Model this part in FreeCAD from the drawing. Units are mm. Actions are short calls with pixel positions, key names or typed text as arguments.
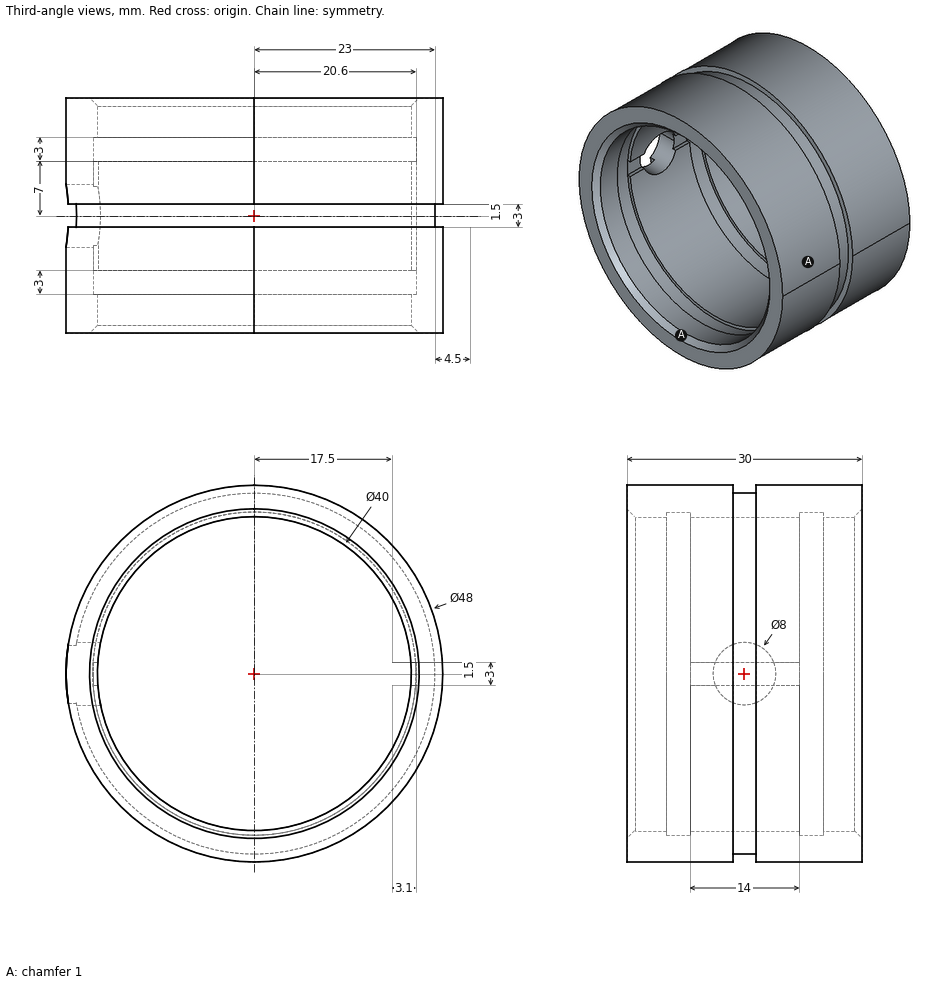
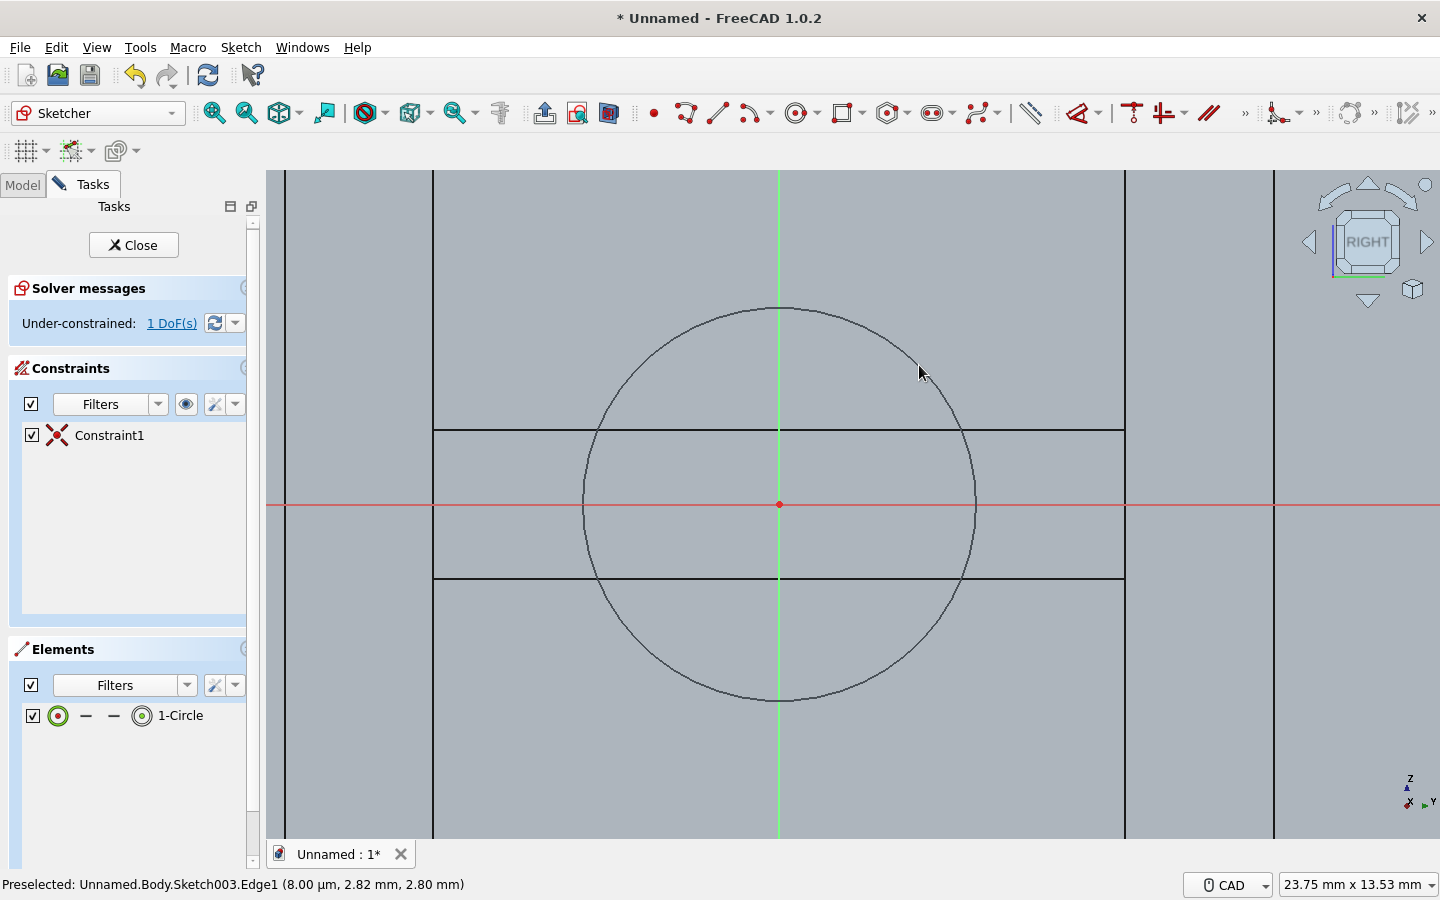
click(1078, 114)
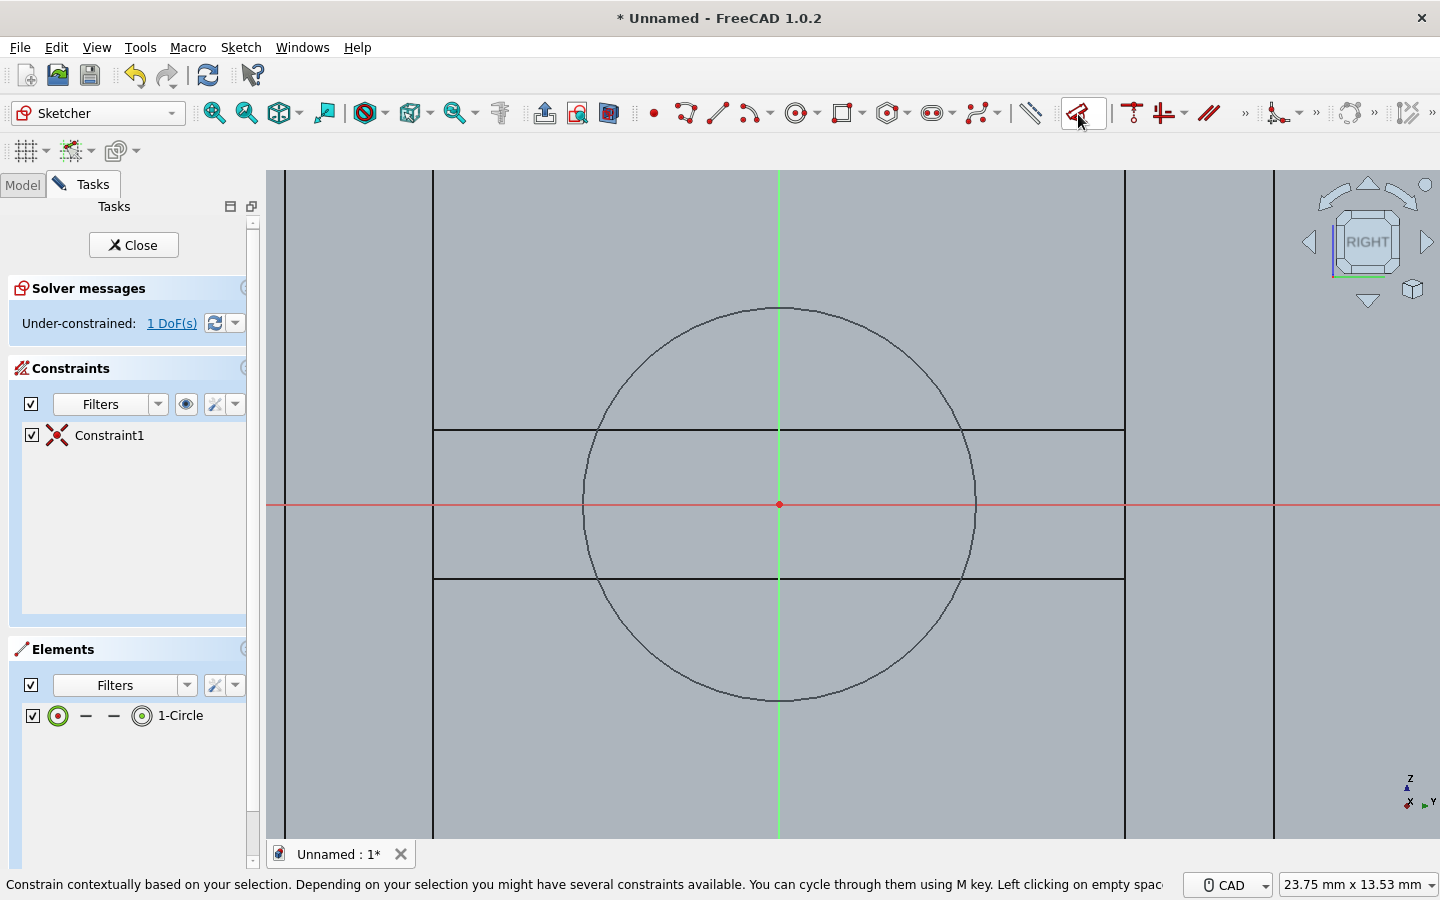
click(918, 365)
click(941, 342)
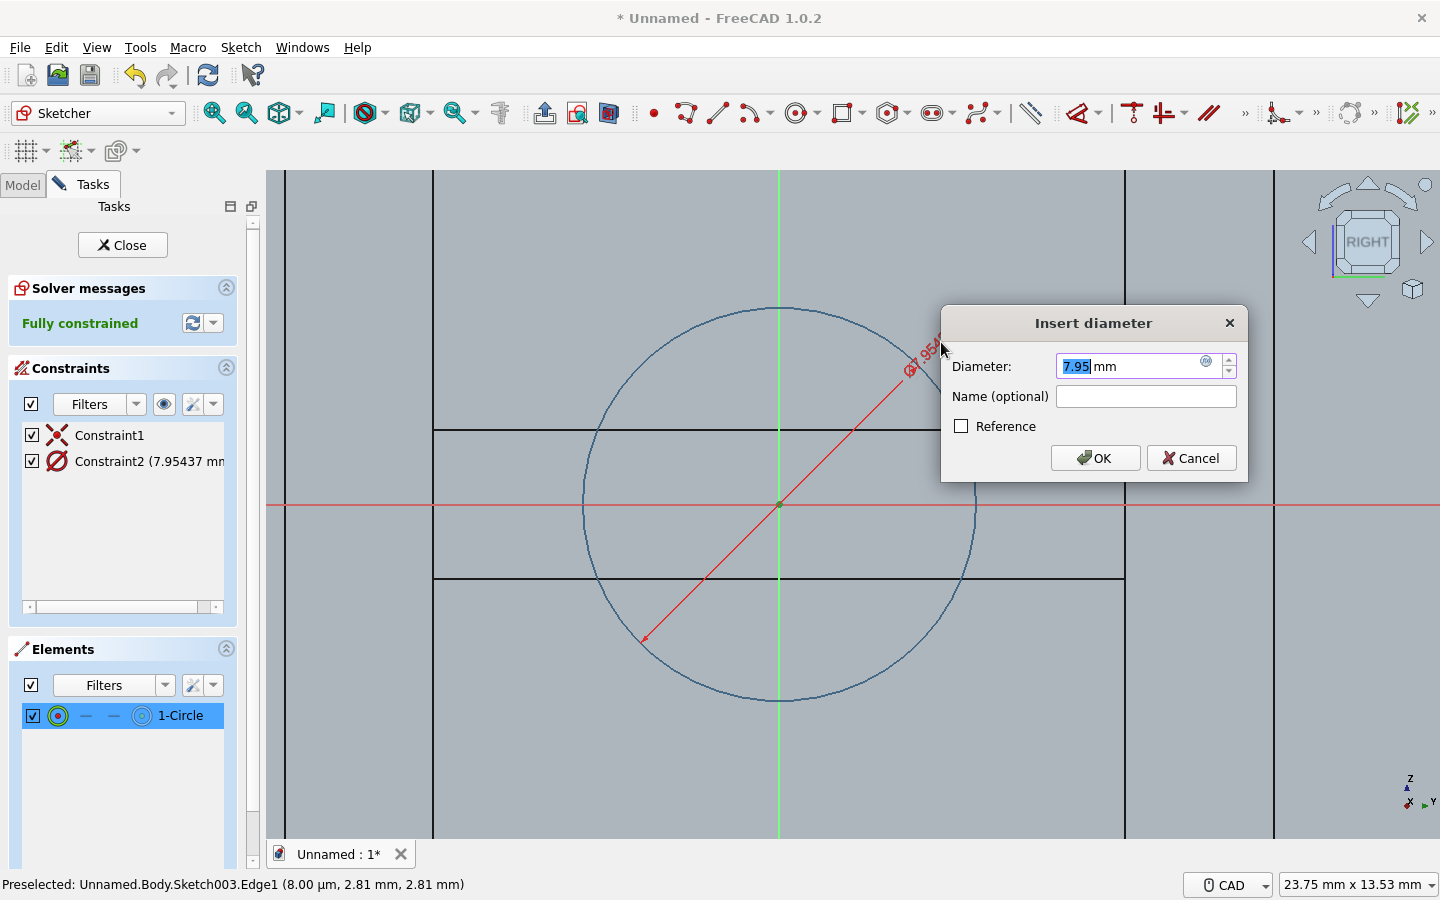
text(8)
key(Return)
key(Escape)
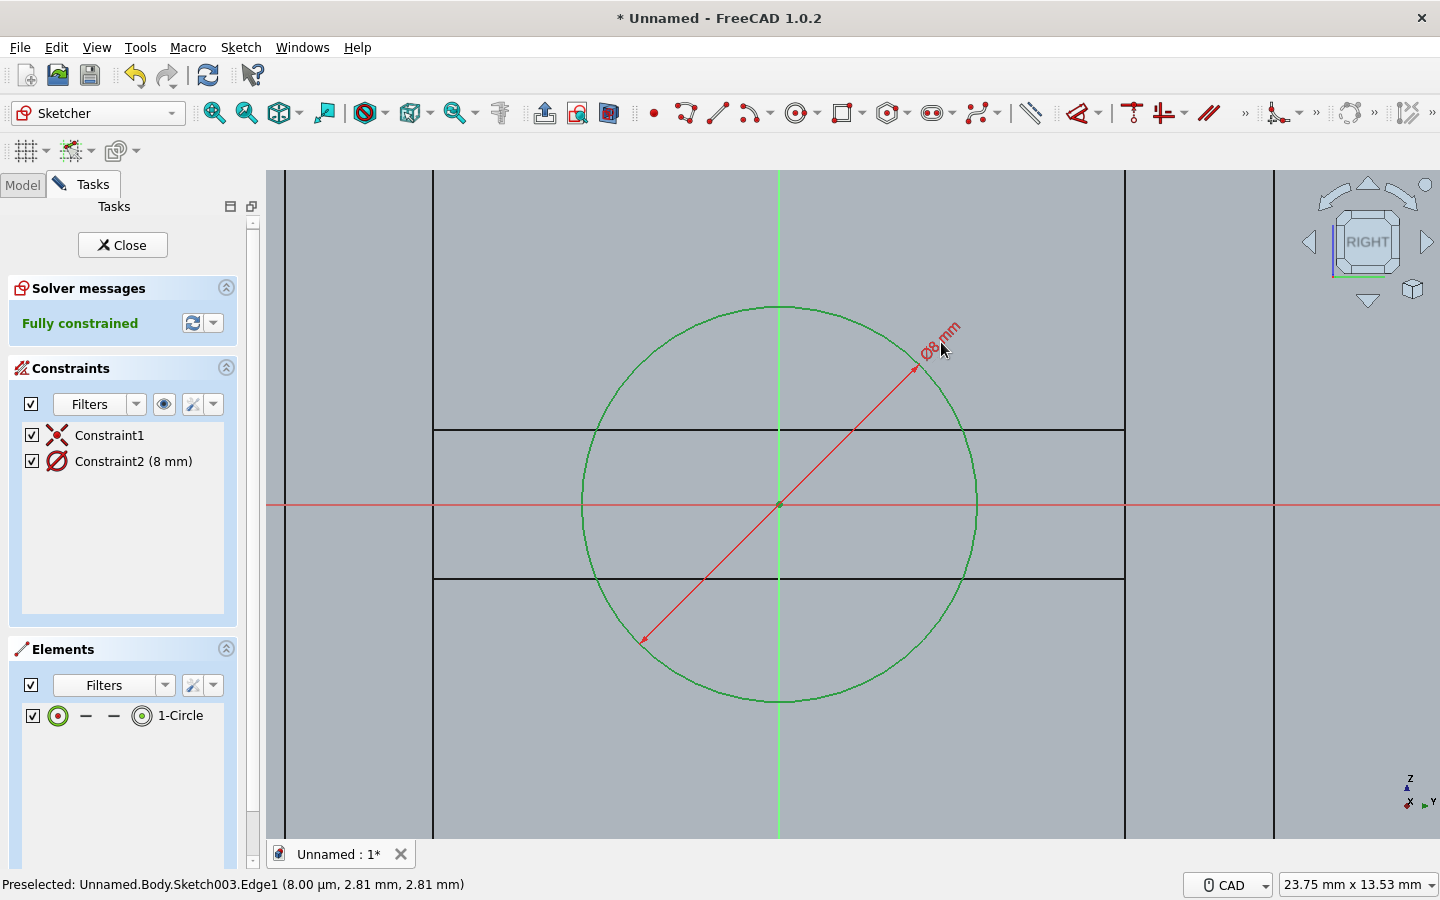
click(123, 245)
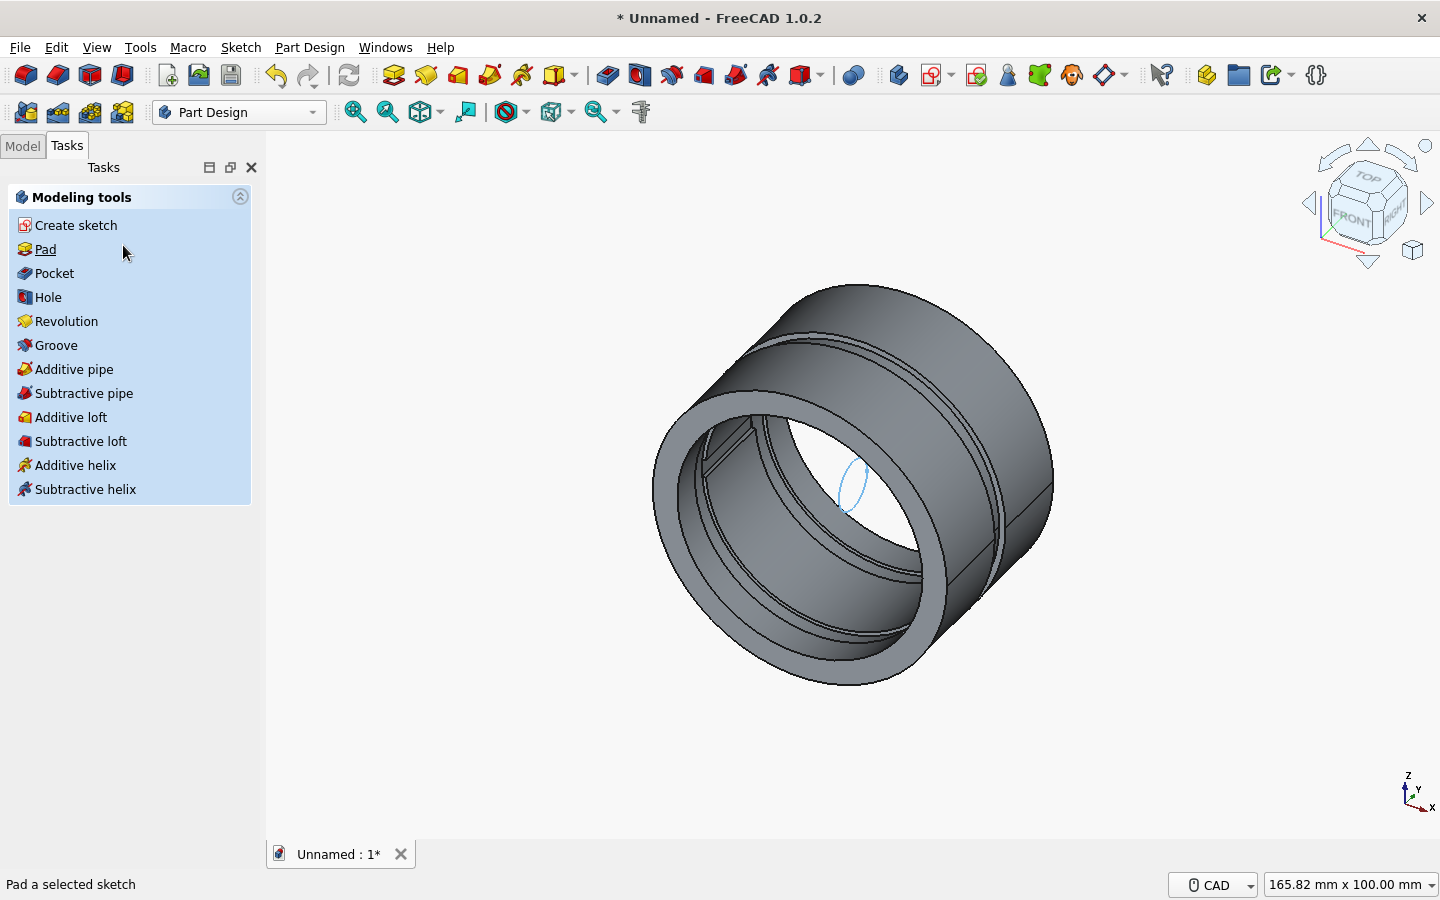
click(608, 76)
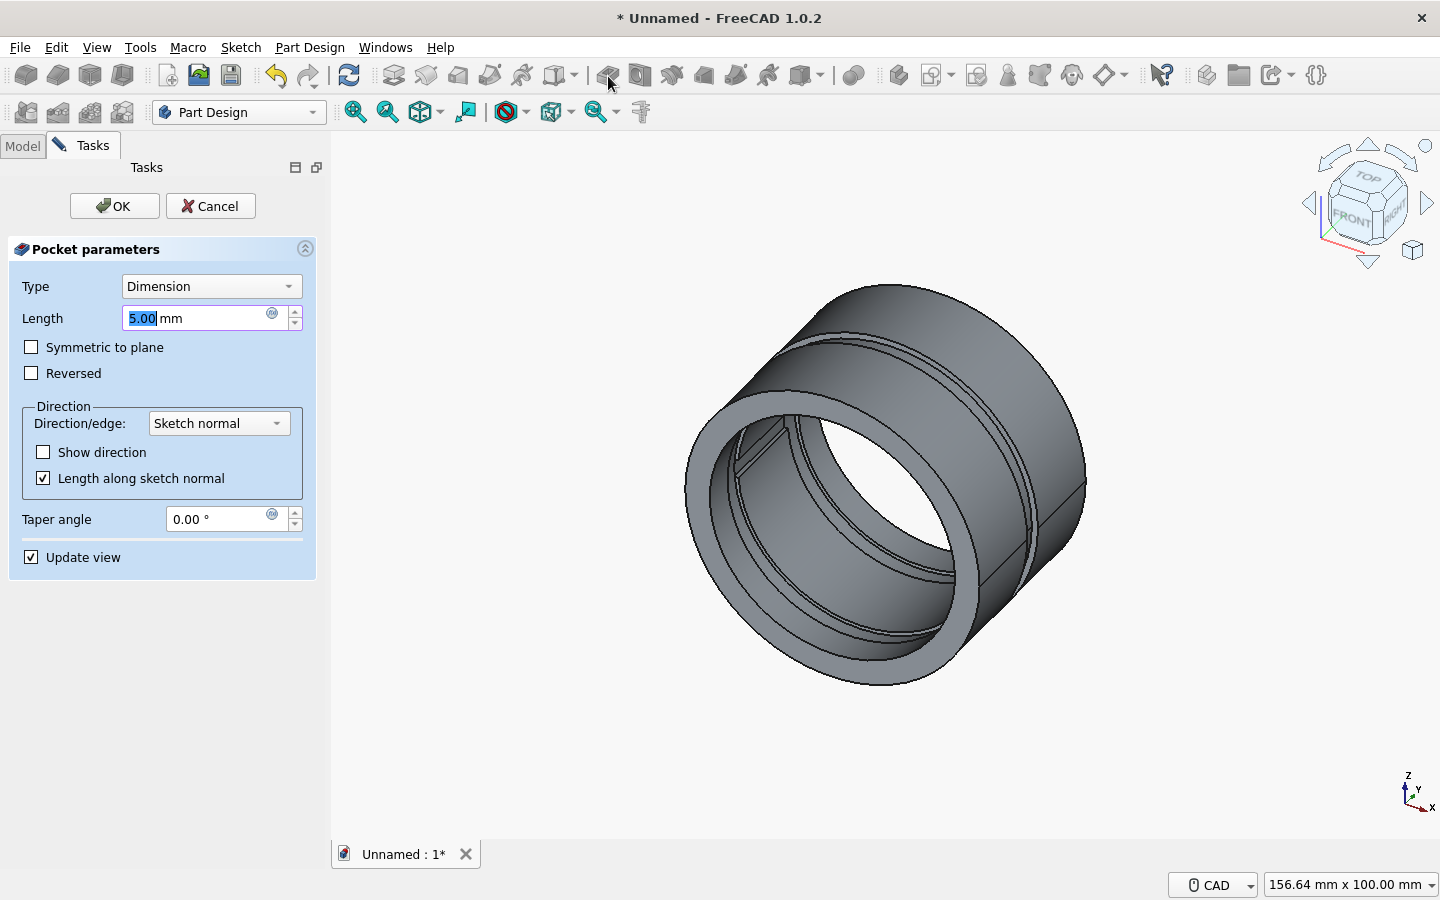
click(212, 286)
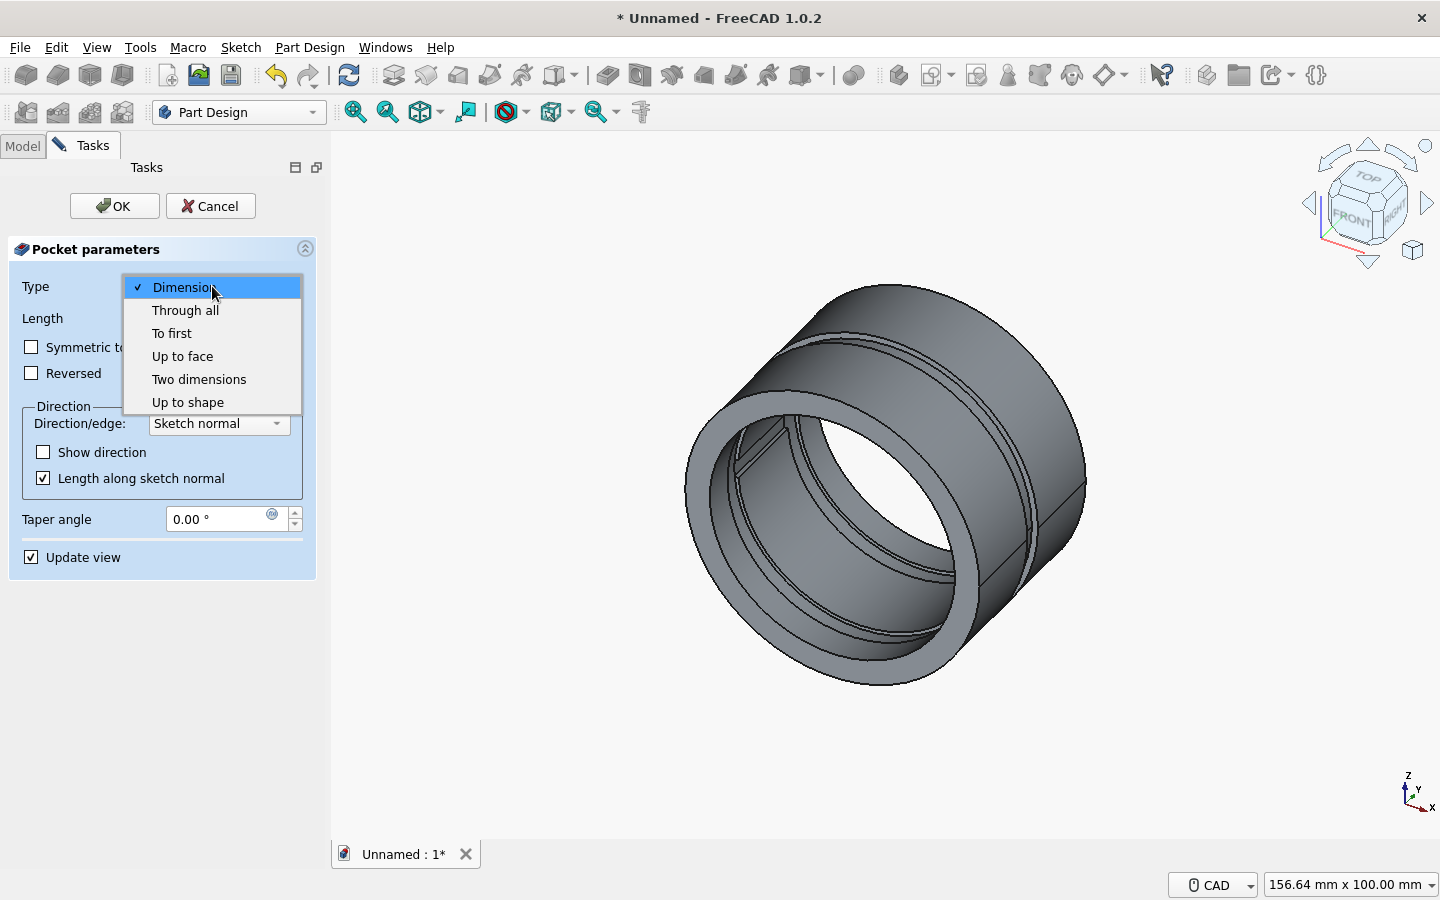
click(212, 310)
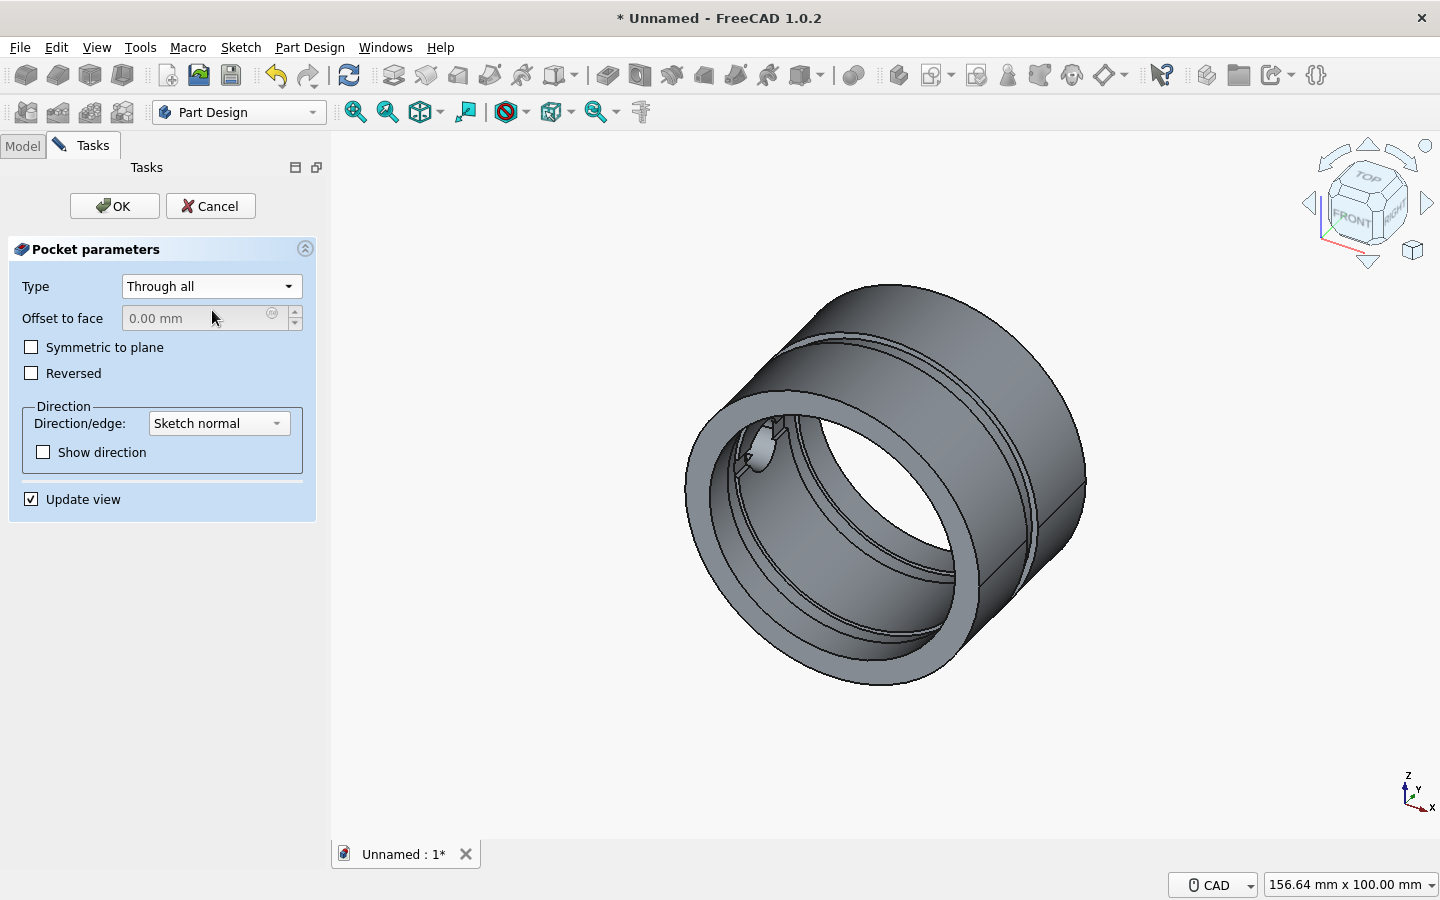
click(115, 206)